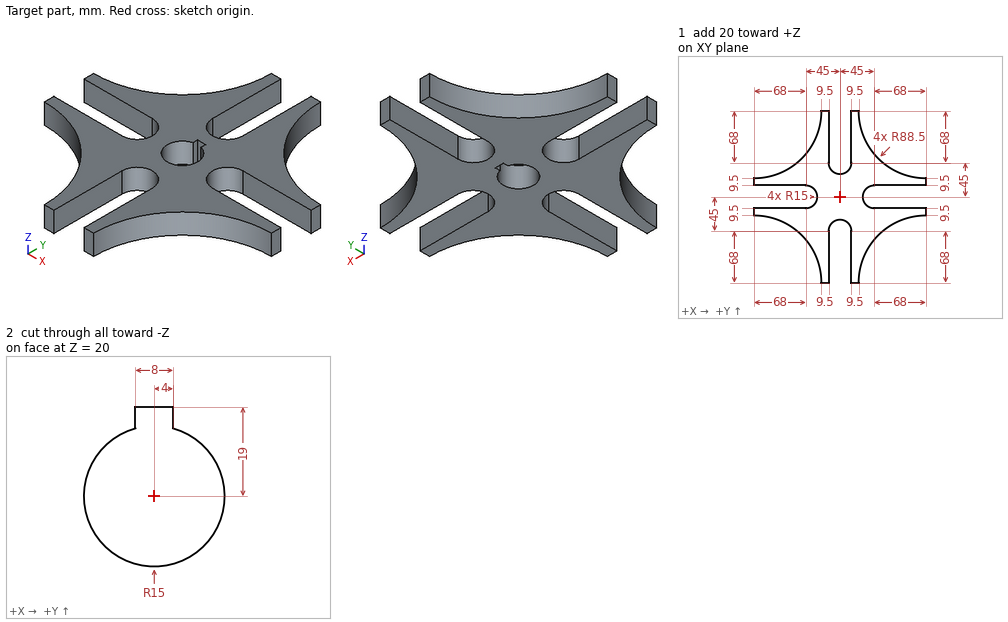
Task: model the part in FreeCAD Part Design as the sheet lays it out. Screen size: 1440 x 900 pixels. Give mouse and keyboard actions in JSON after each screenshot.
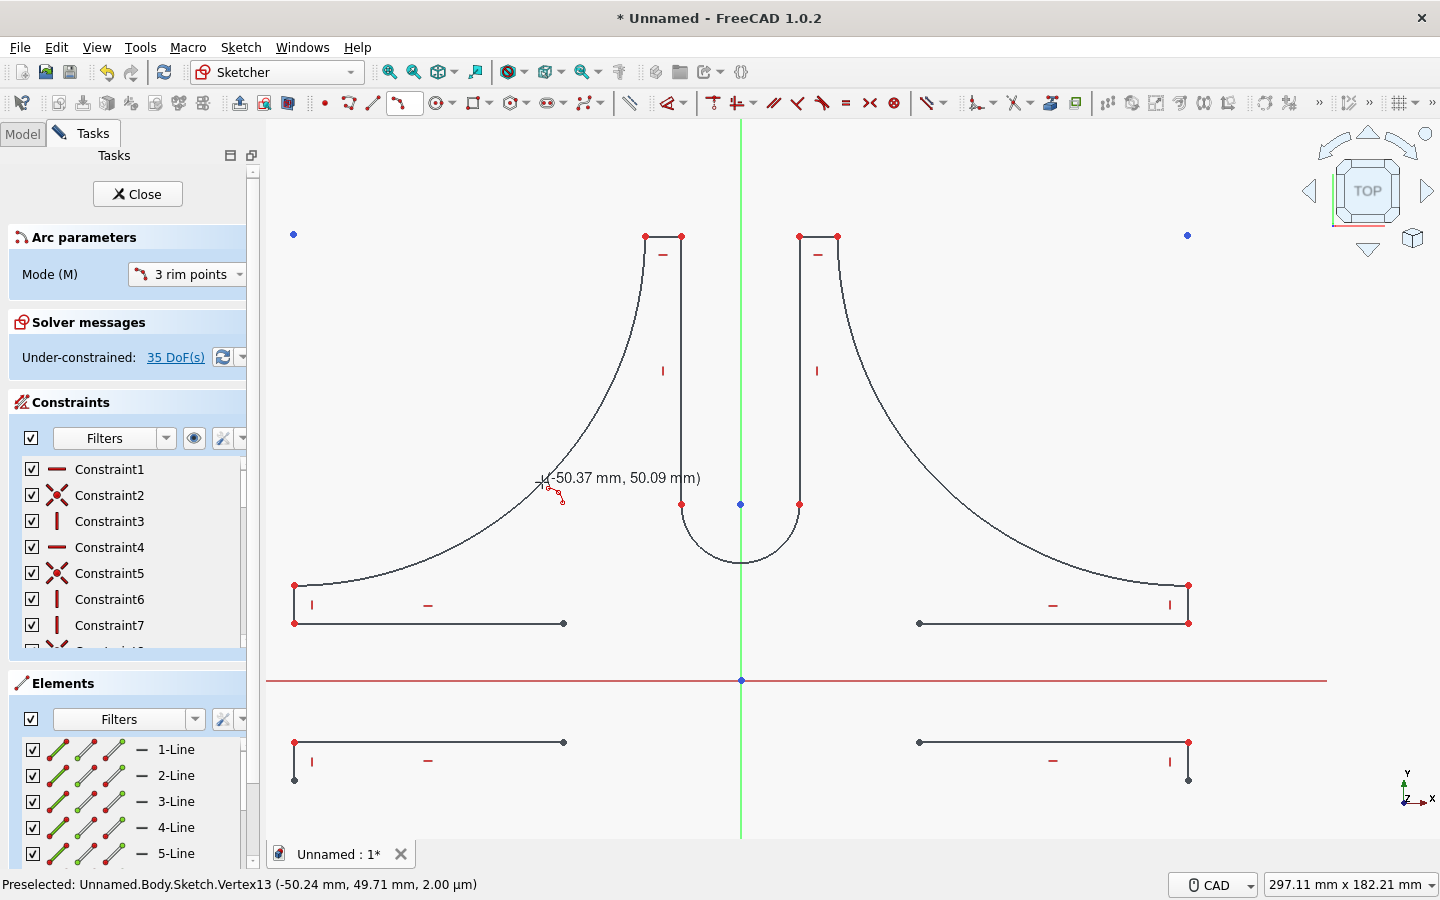
{"action": "left_click", "coordinate": [563, 624]}
{"action": "left_click", "coordinate": [563, 742]}
{"action": "left_click", "coordinate": [611, 716]}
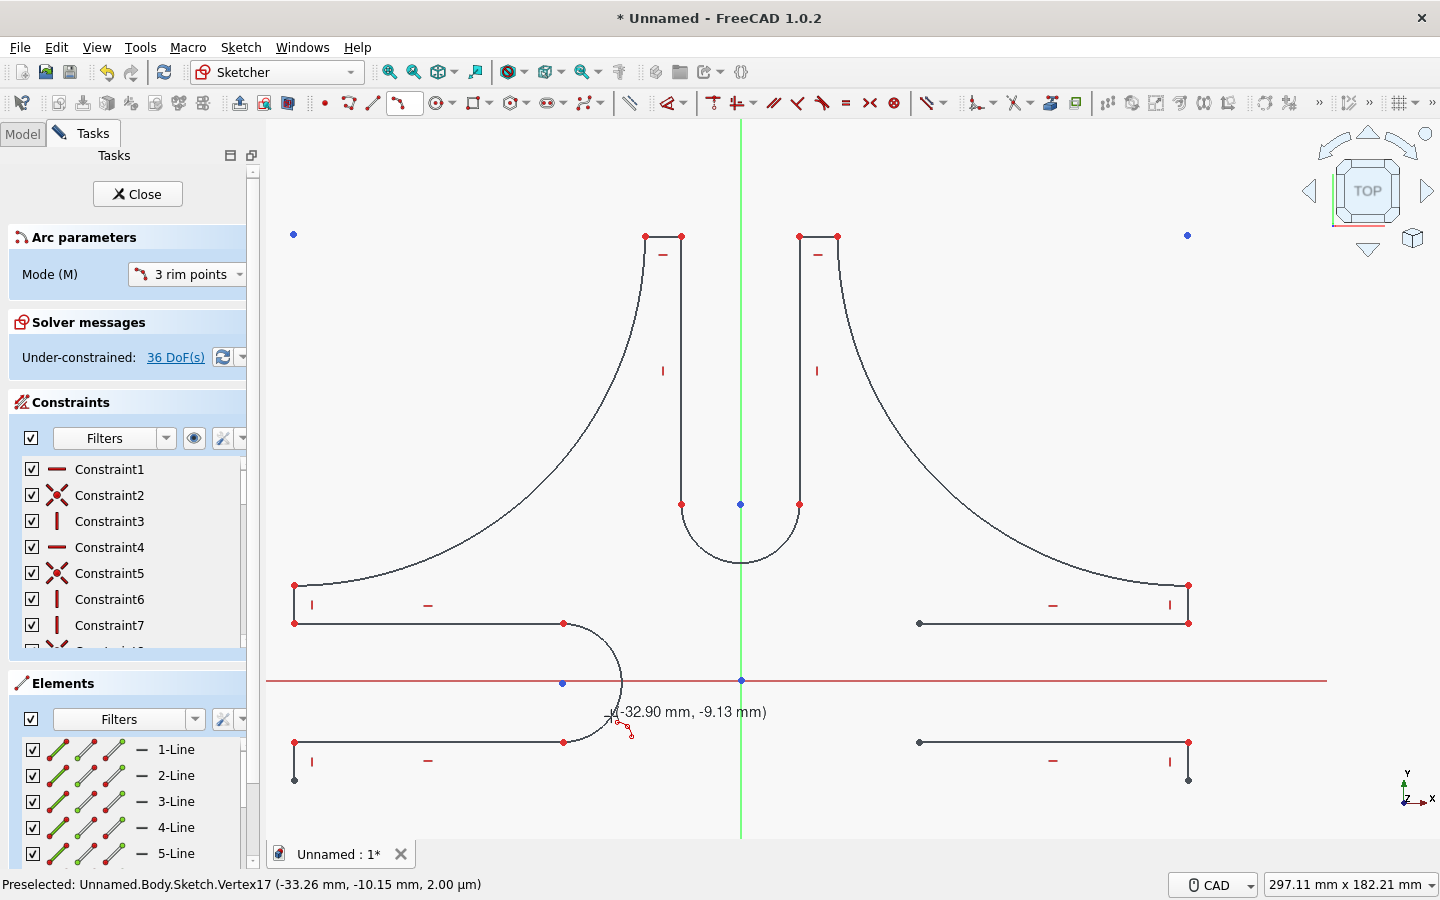
{"action": "left_click", "coordinate": [294, 780]}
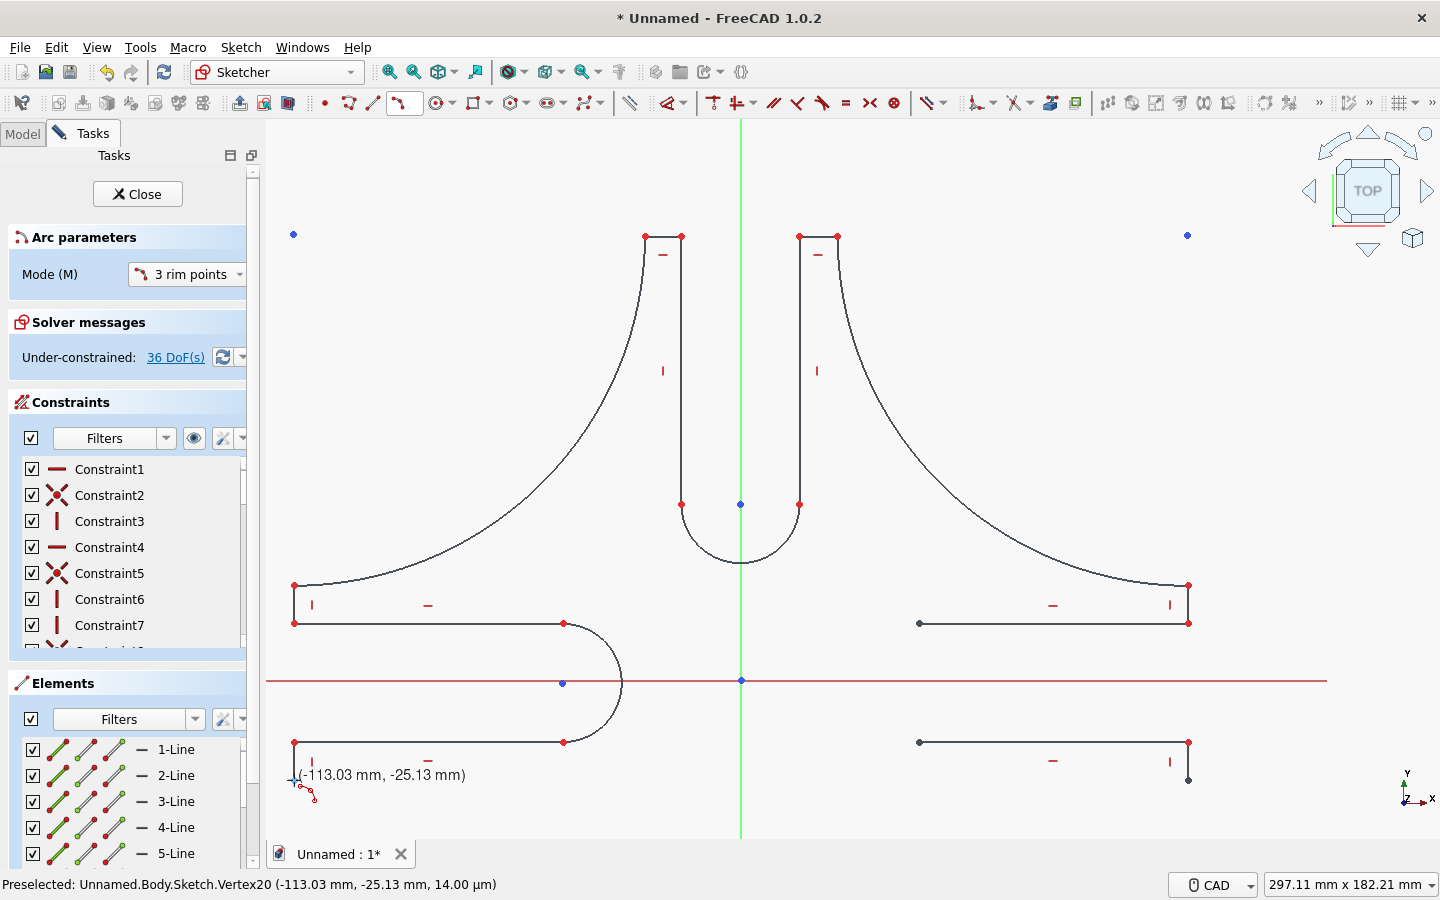
{"action": "scroll", "coordinate": [837, 233], "scroll_direction": "down", "scroll_amount": 3}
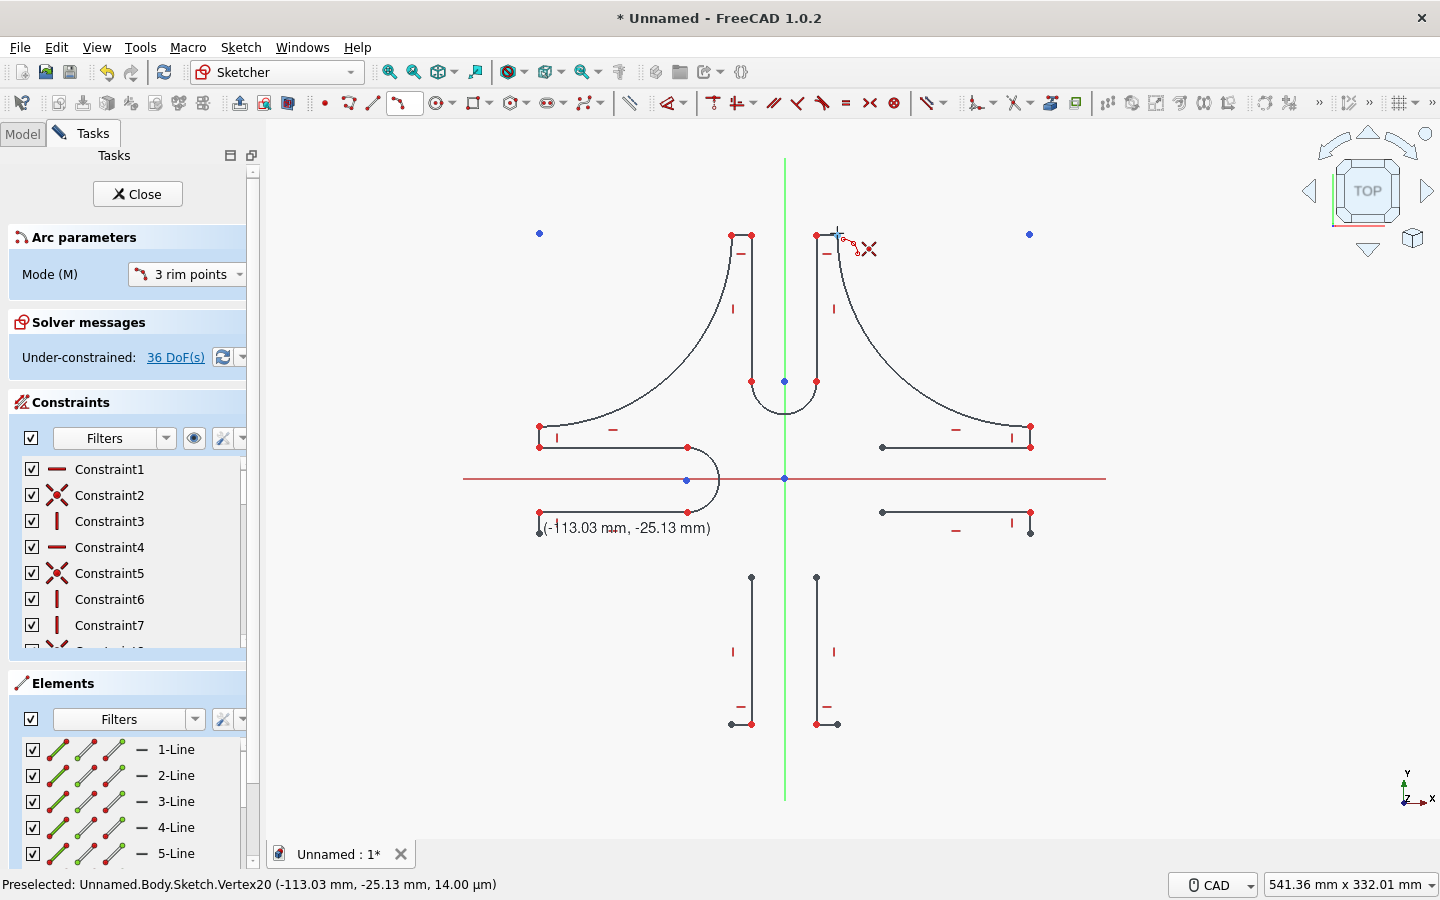
{"action": "scroll", "coordinate": [731, 724], "scroll_direction": "up", "scroll_amount": 3}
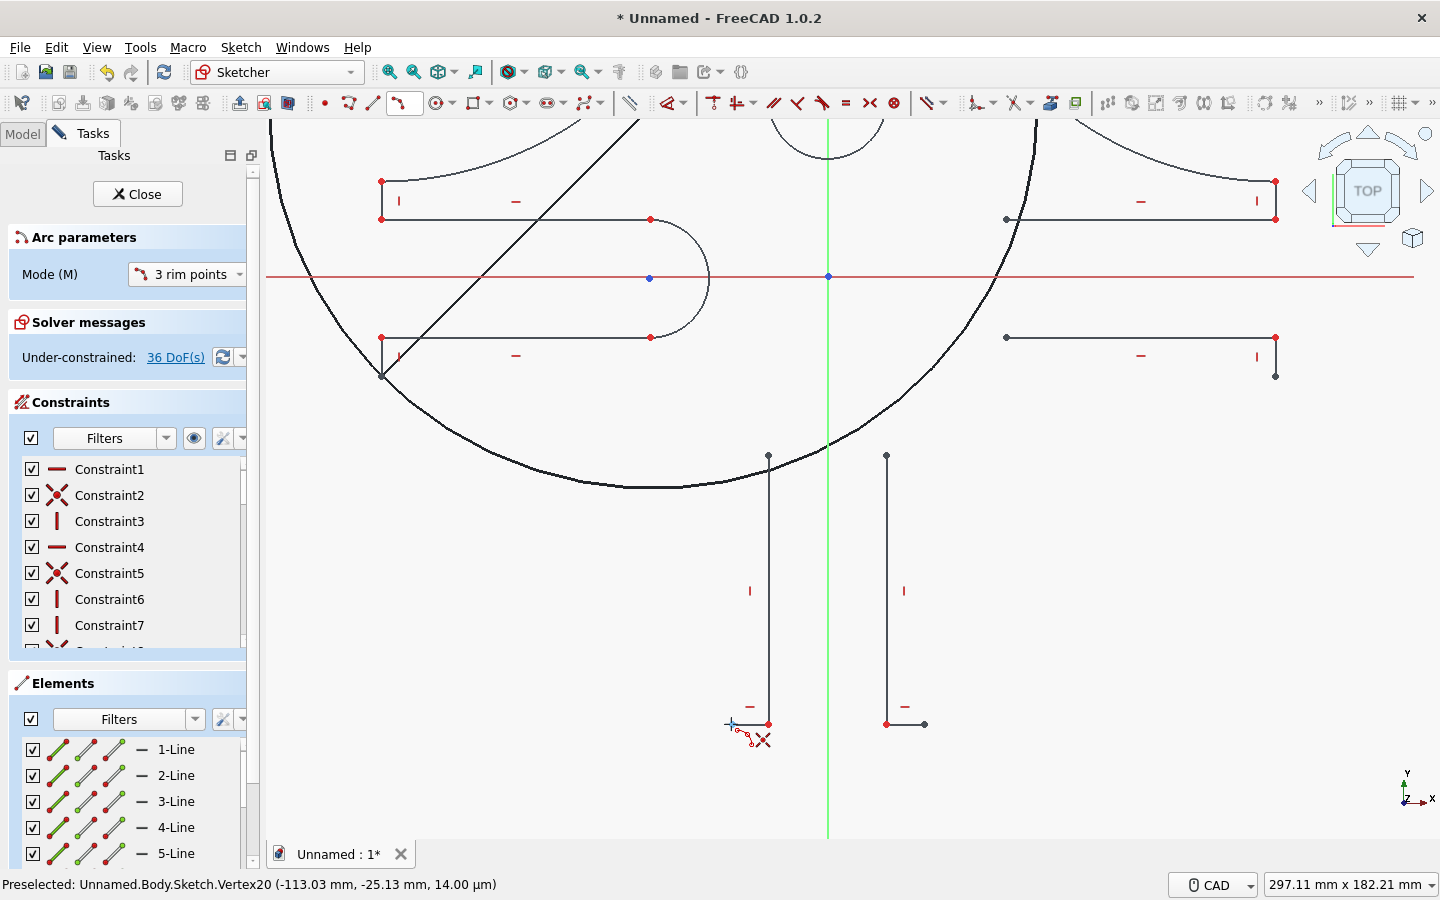
{"action": "left_click", "coordinate": [732, 725]}
{"action": "left_click", "coordinate": [629, 476]}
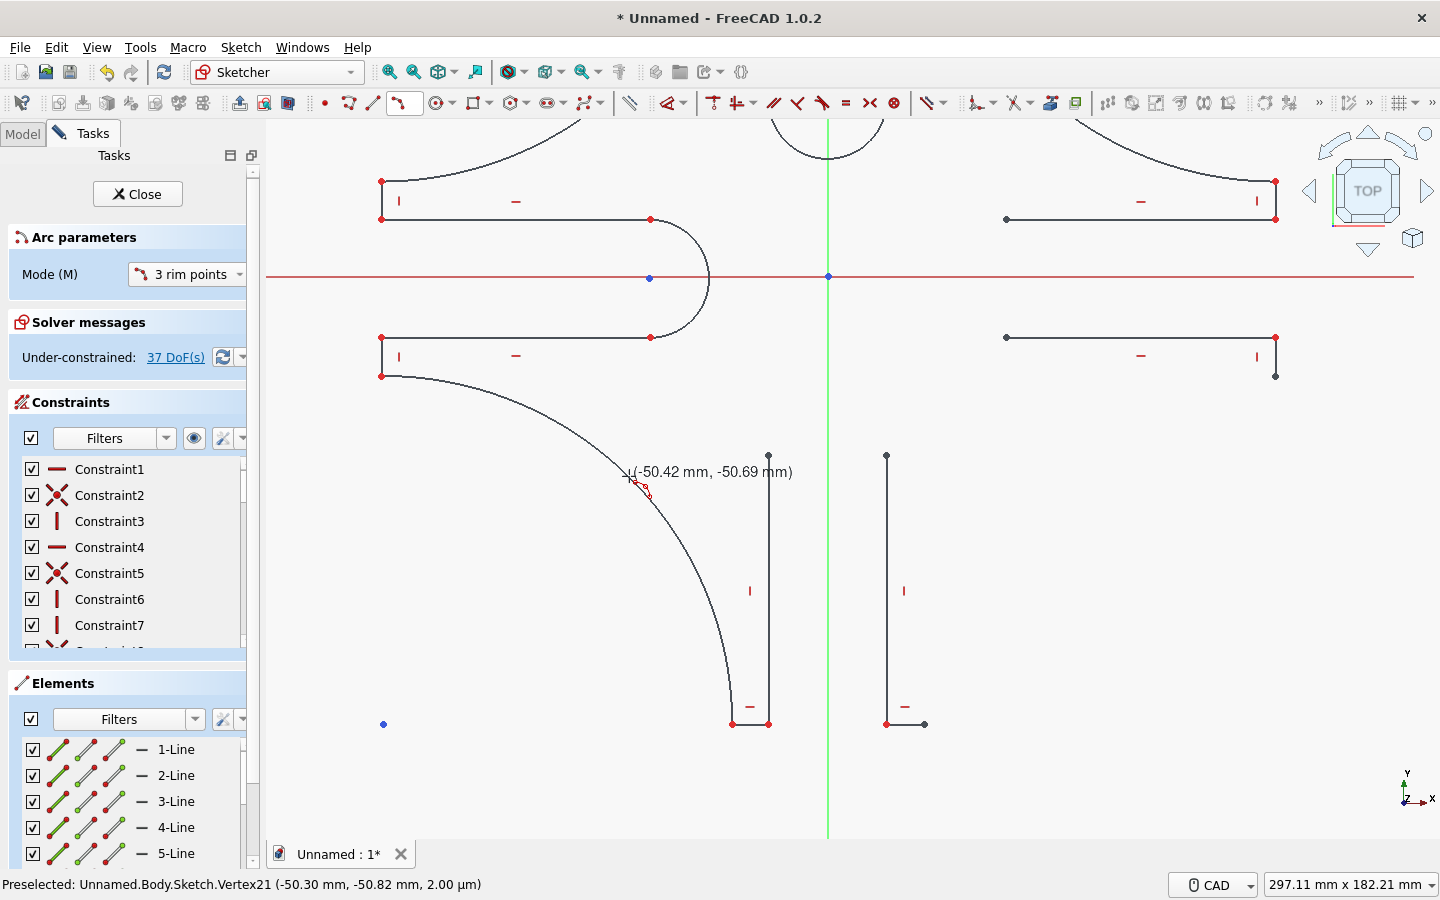
{"action": "left_click", "coordinate": [769, 456]}
{"action": "left_click", "coordinate": [887, 456]}
{"action": "left_click", "coordinate": [863, 407]}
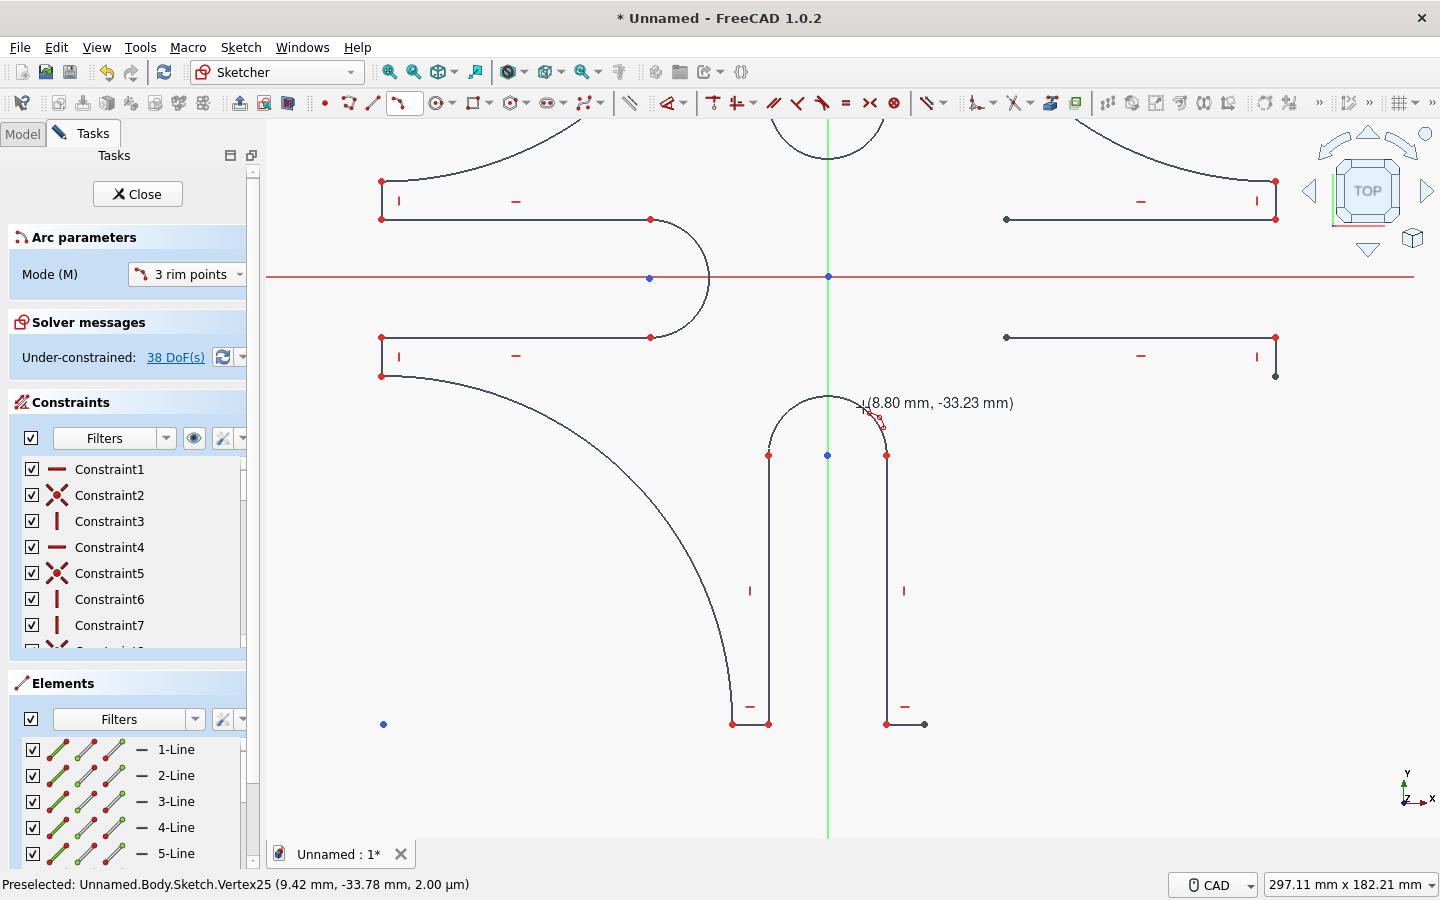
{"action": "left_click", "coordinate": [925, 725]}
{"action": "left_click", "coordinate": [1276, 376]}
{"action": "left_click", "coordinate": [1027, 476]}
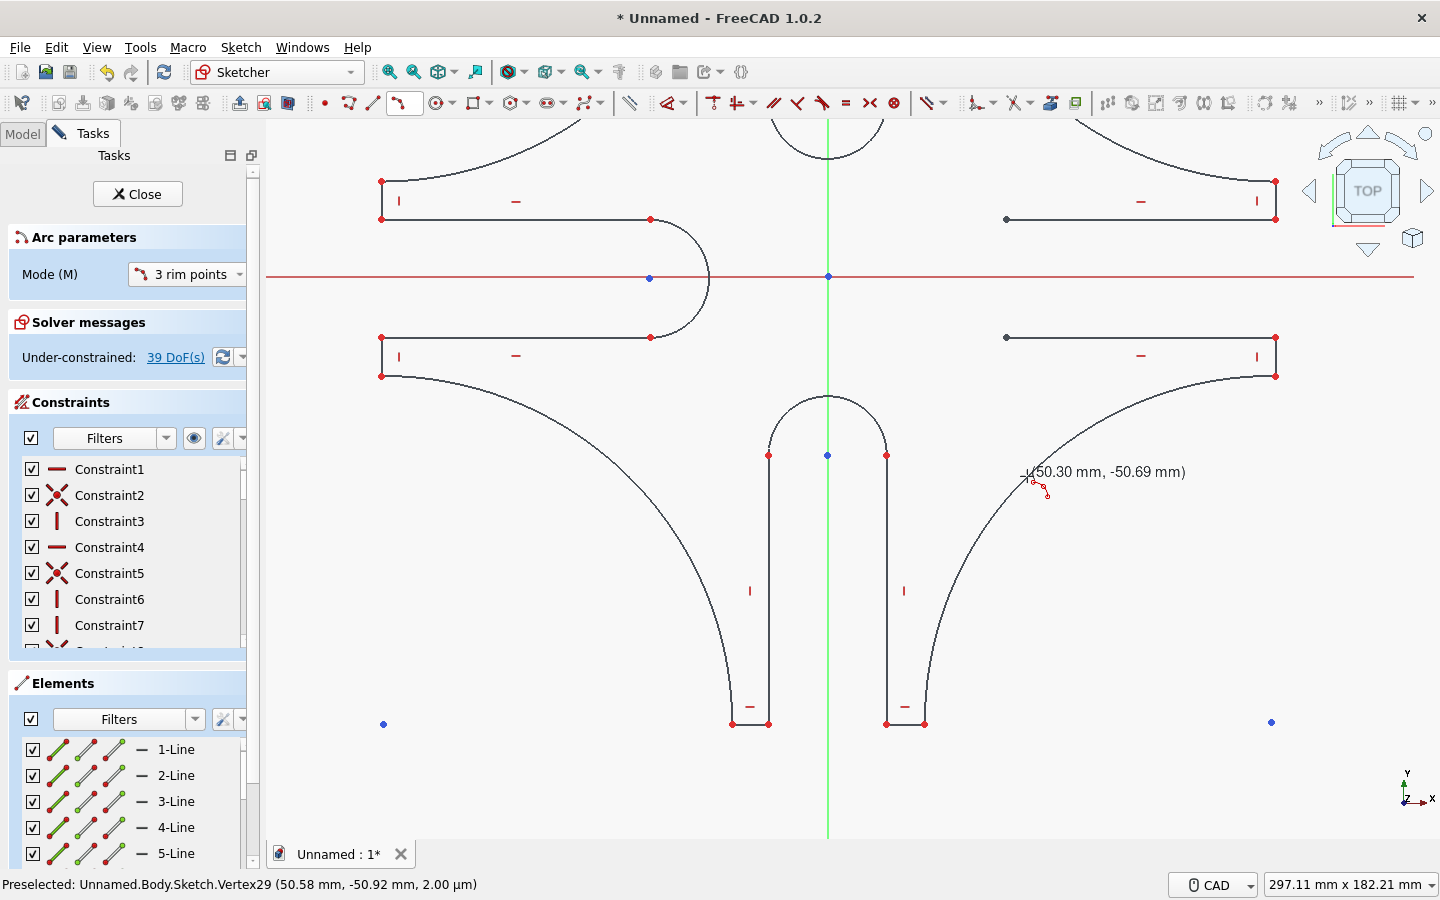
{"action": "left_click", "coordinate": [1007, 338]}
{"action": "left_click", "coordinate": [1007, 220]}
{"action": "left_click", "coordinate": [958, 242]}
{"action": "key", "text": "Escape"}